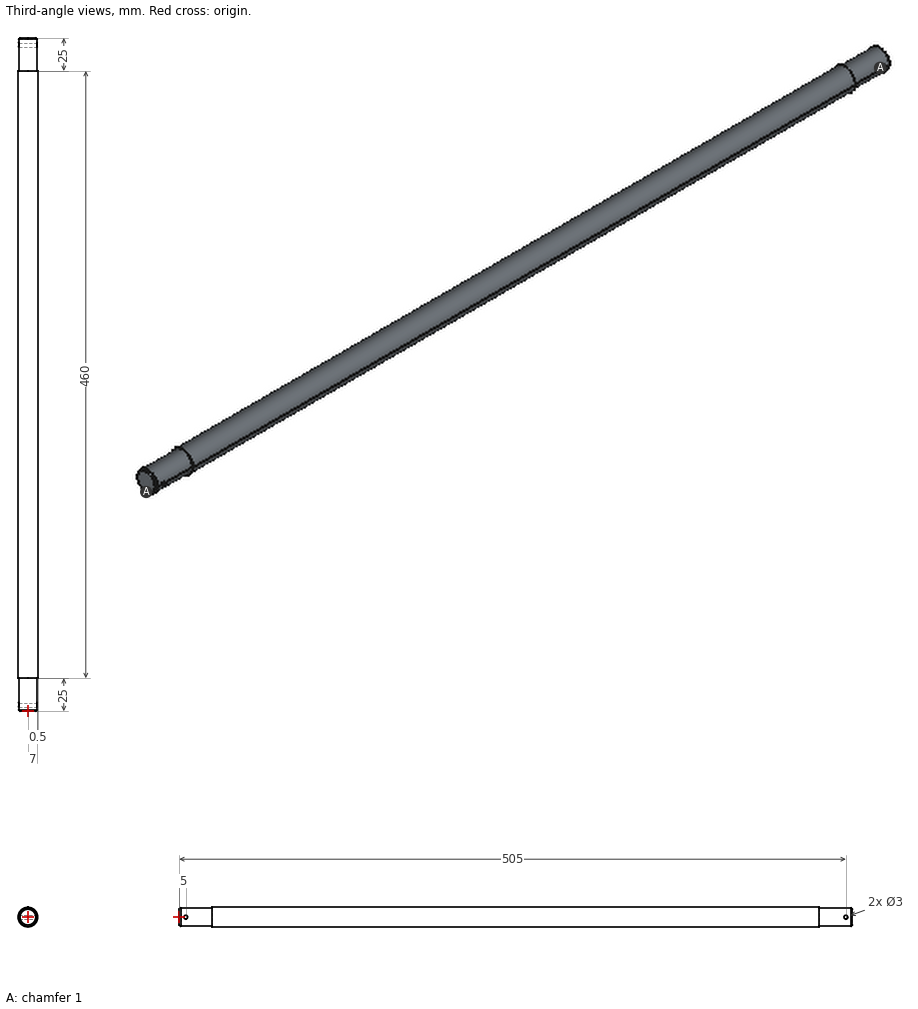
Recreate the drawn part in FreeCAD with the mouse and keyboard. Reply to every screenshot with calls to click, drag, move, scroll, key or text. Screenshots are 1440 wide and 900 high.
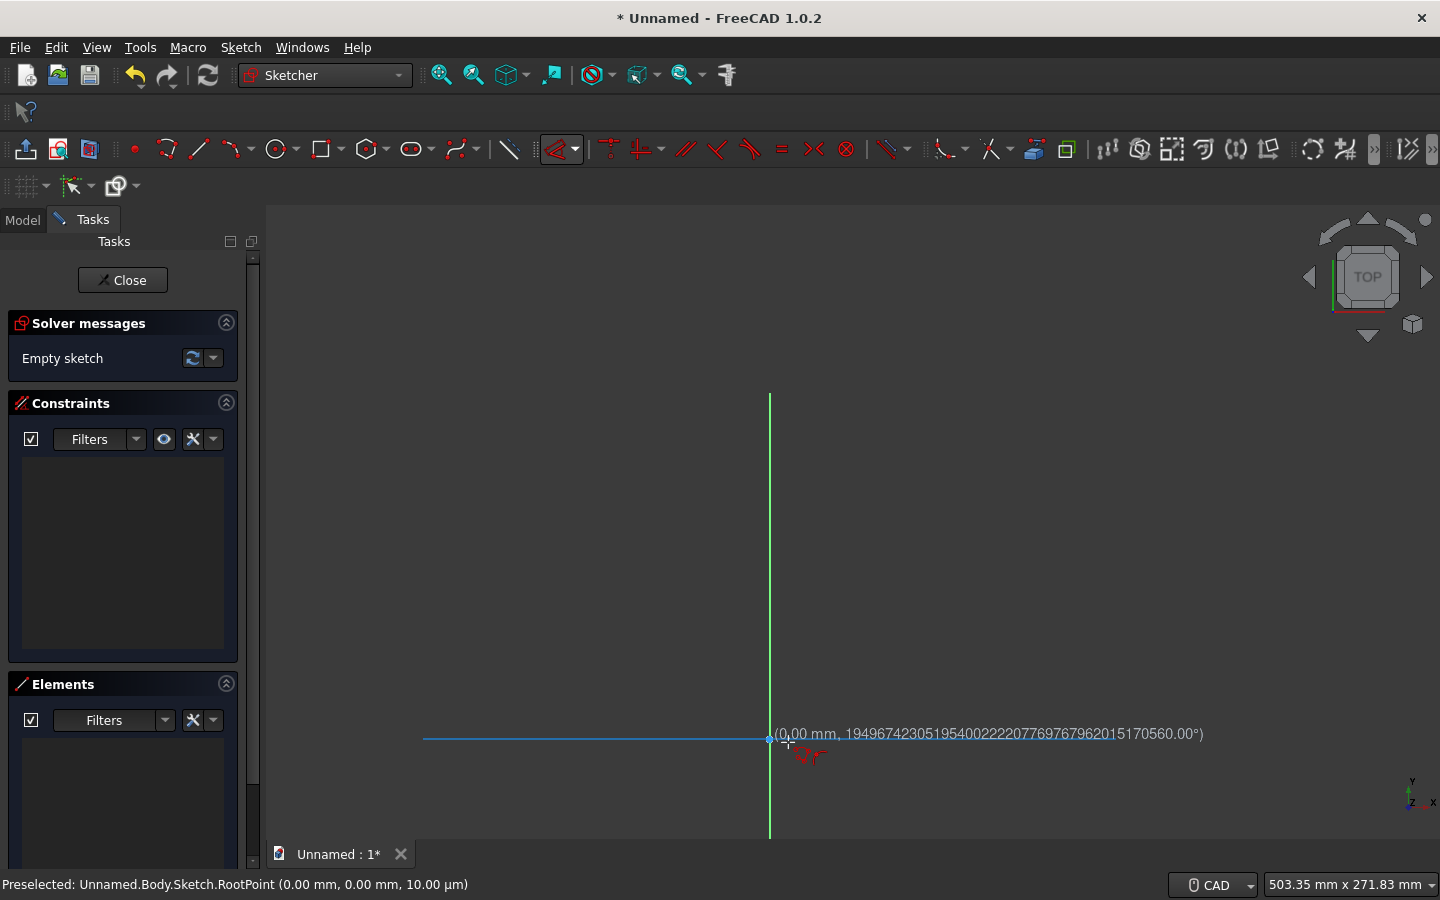
click(786, 730)
click(786, 681)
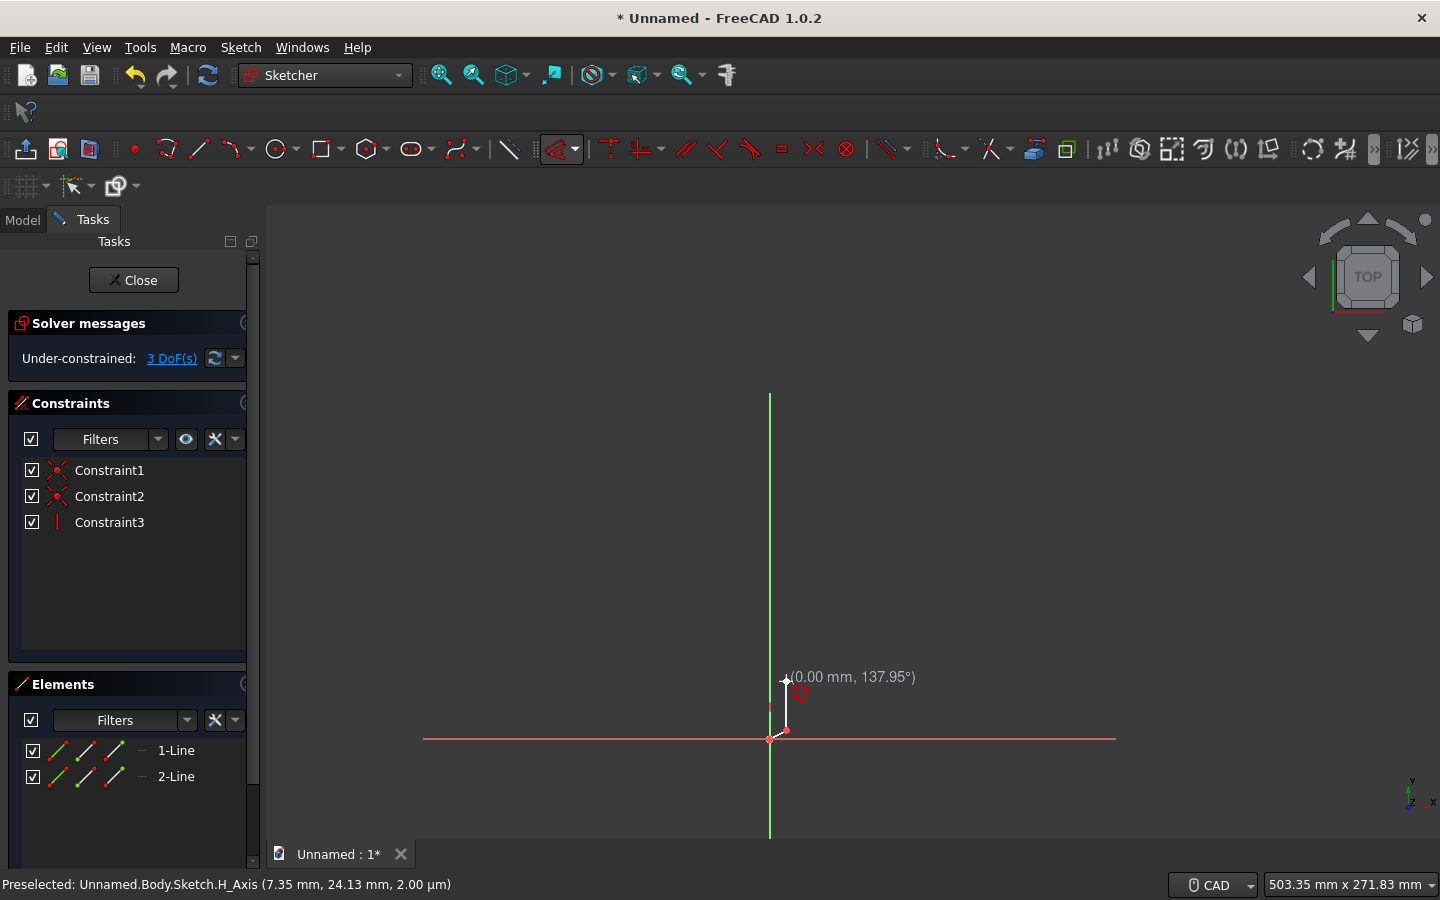
scroll(787, 681, up, 14)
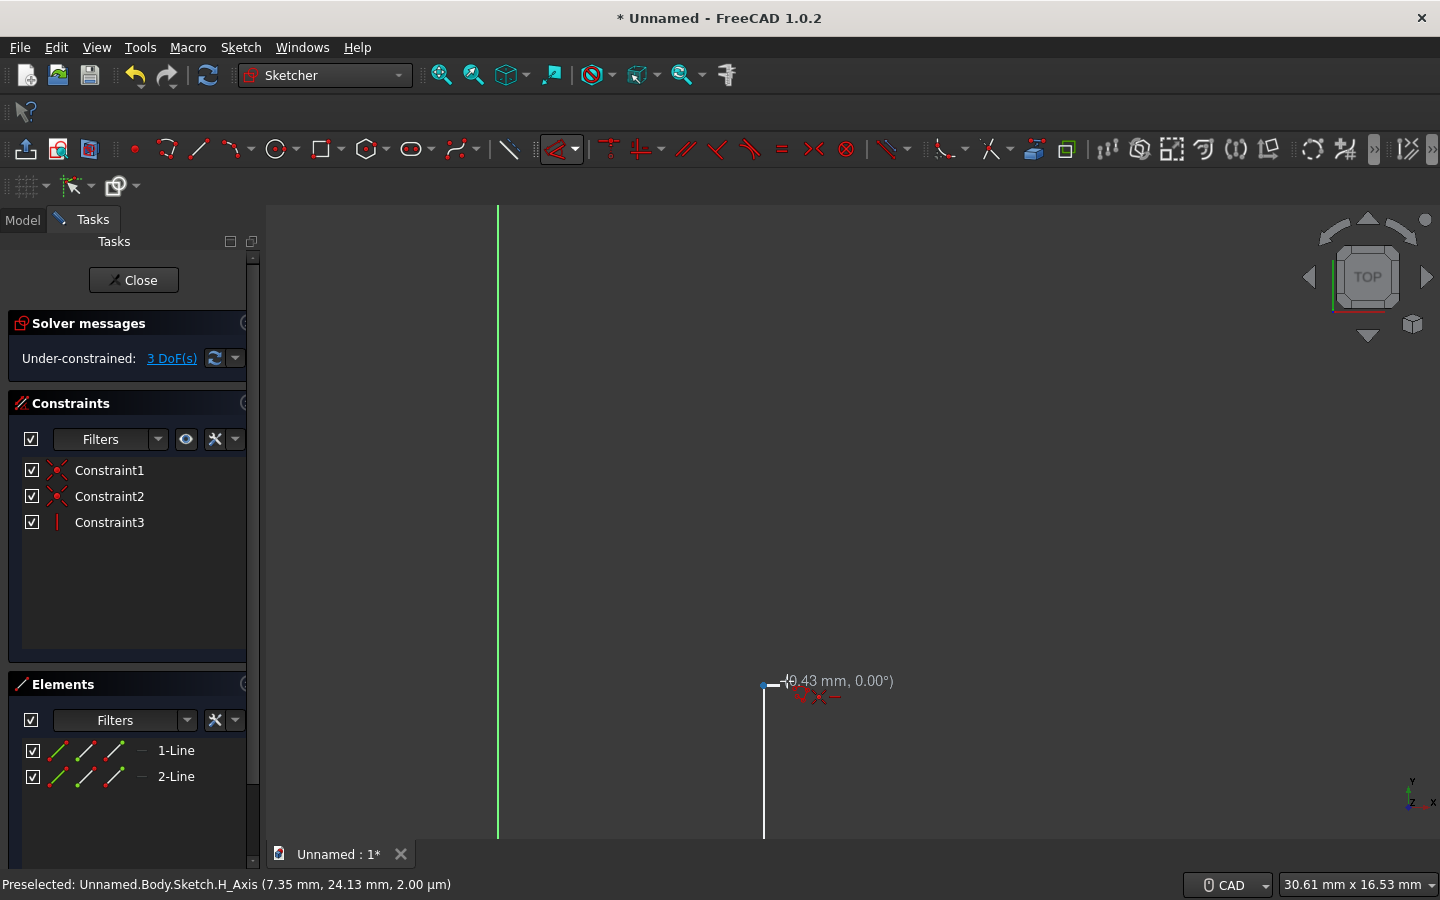
click(786, 669)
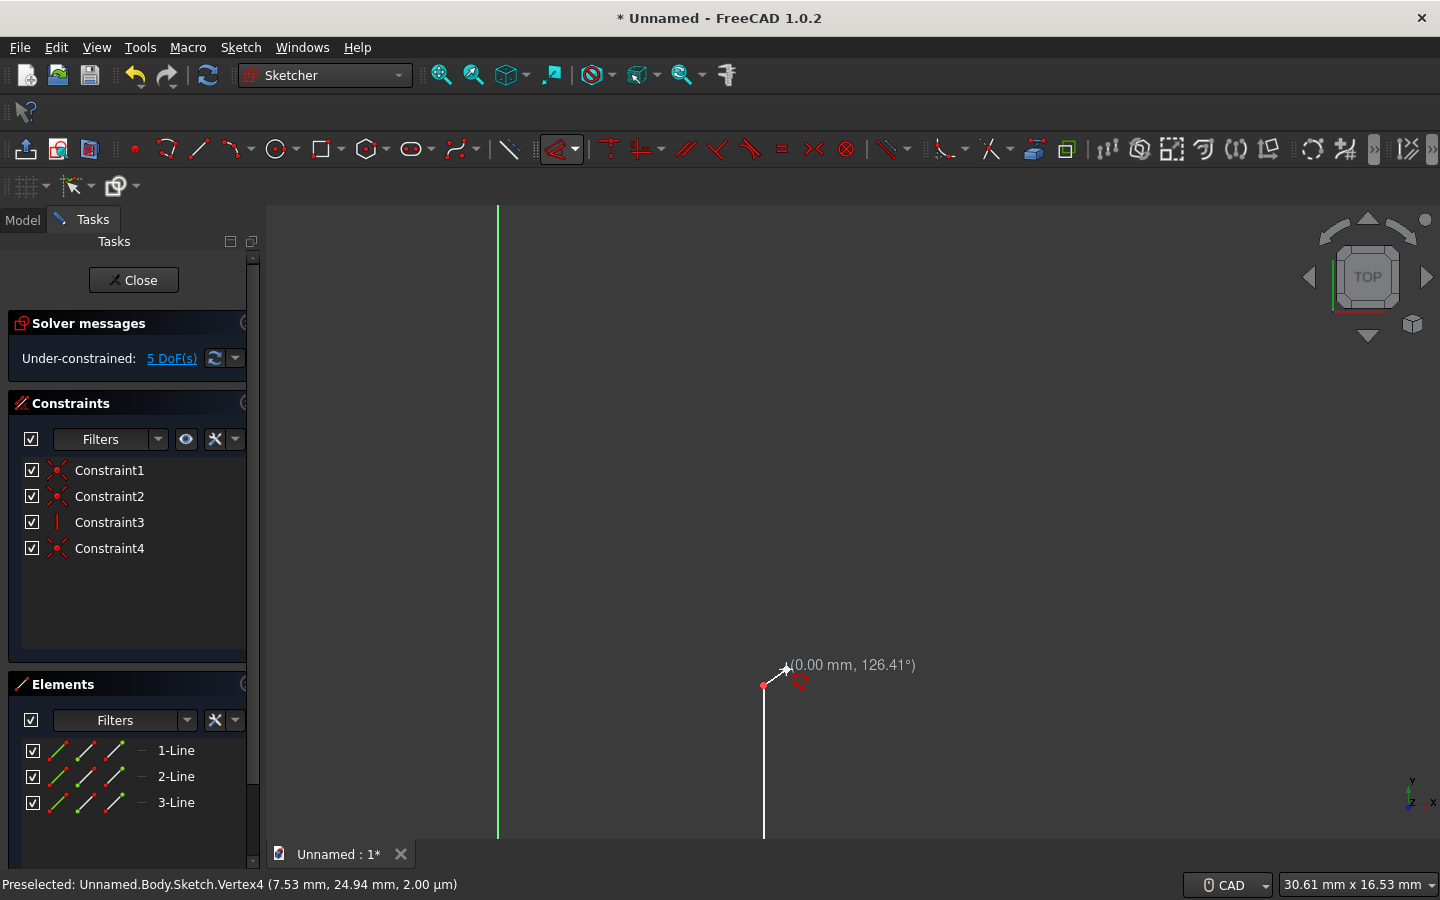
scroll(784, 522, down, 15)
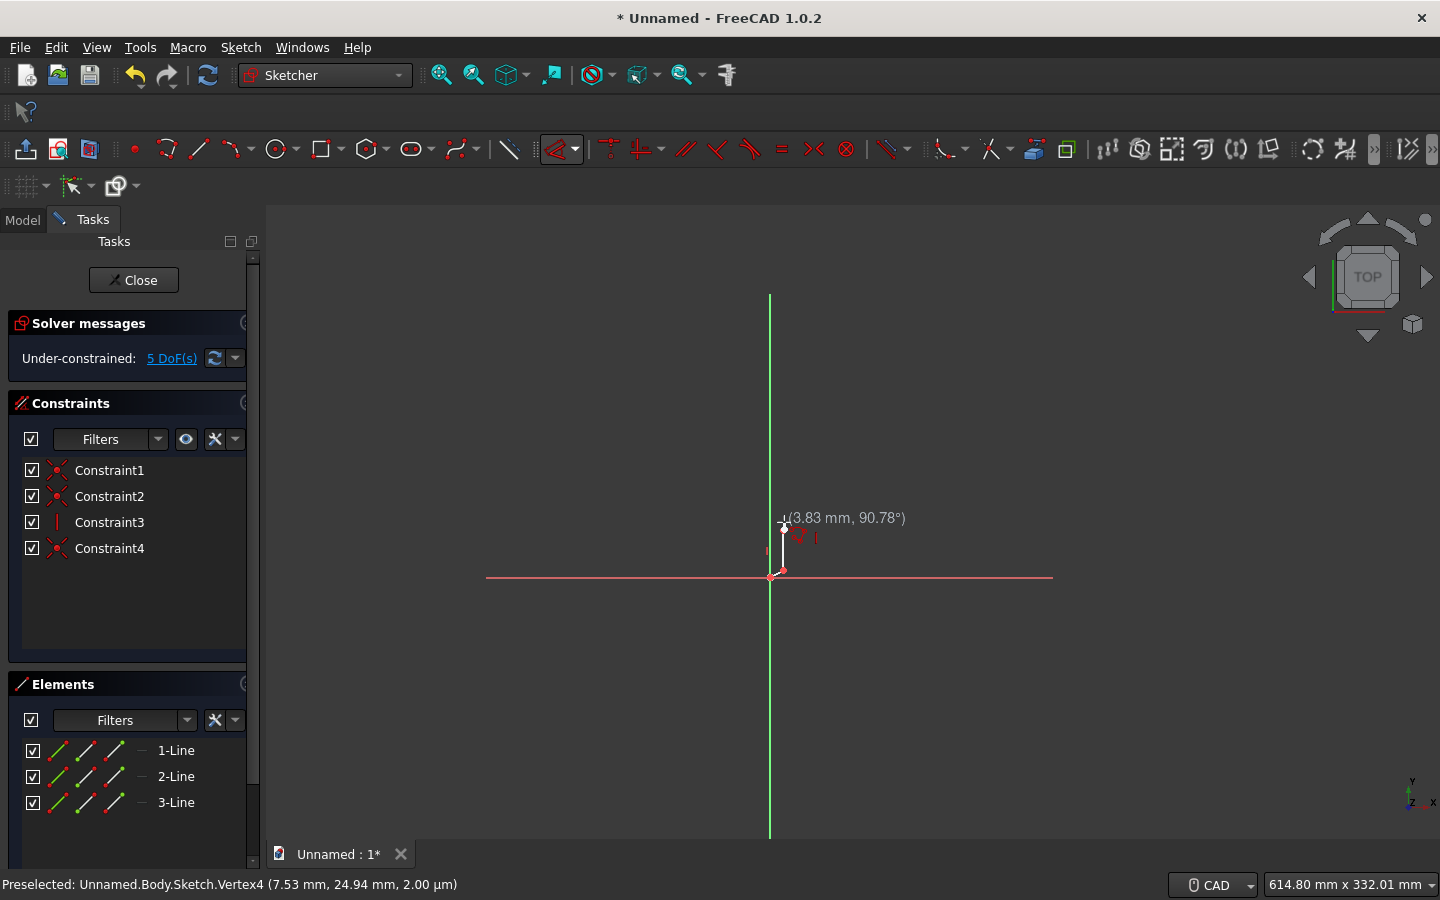
scroll(790, 811, down, 4)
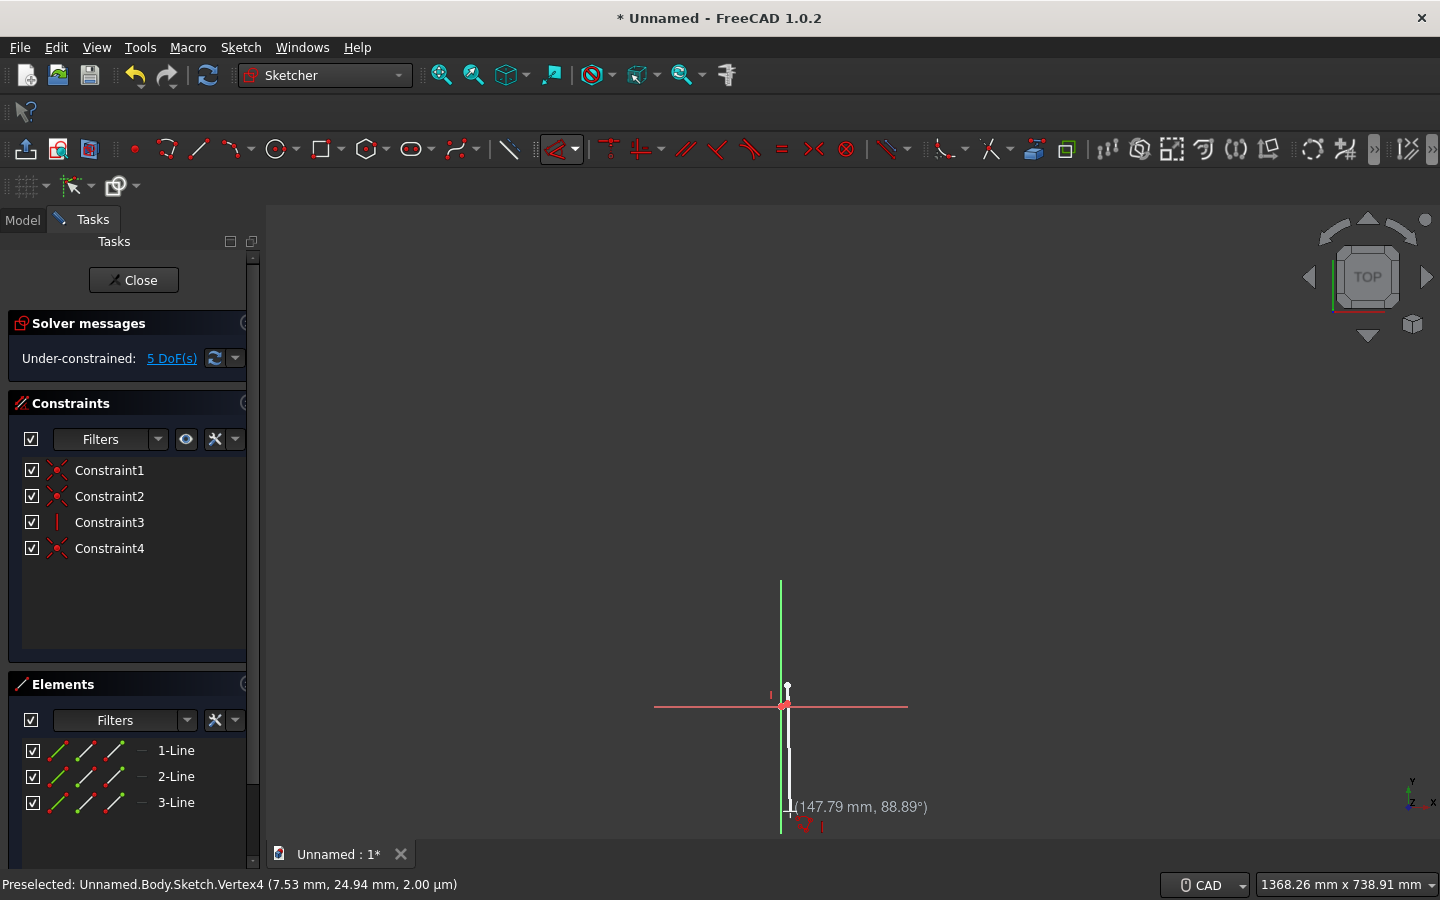
scroll(788, 290, up, 5)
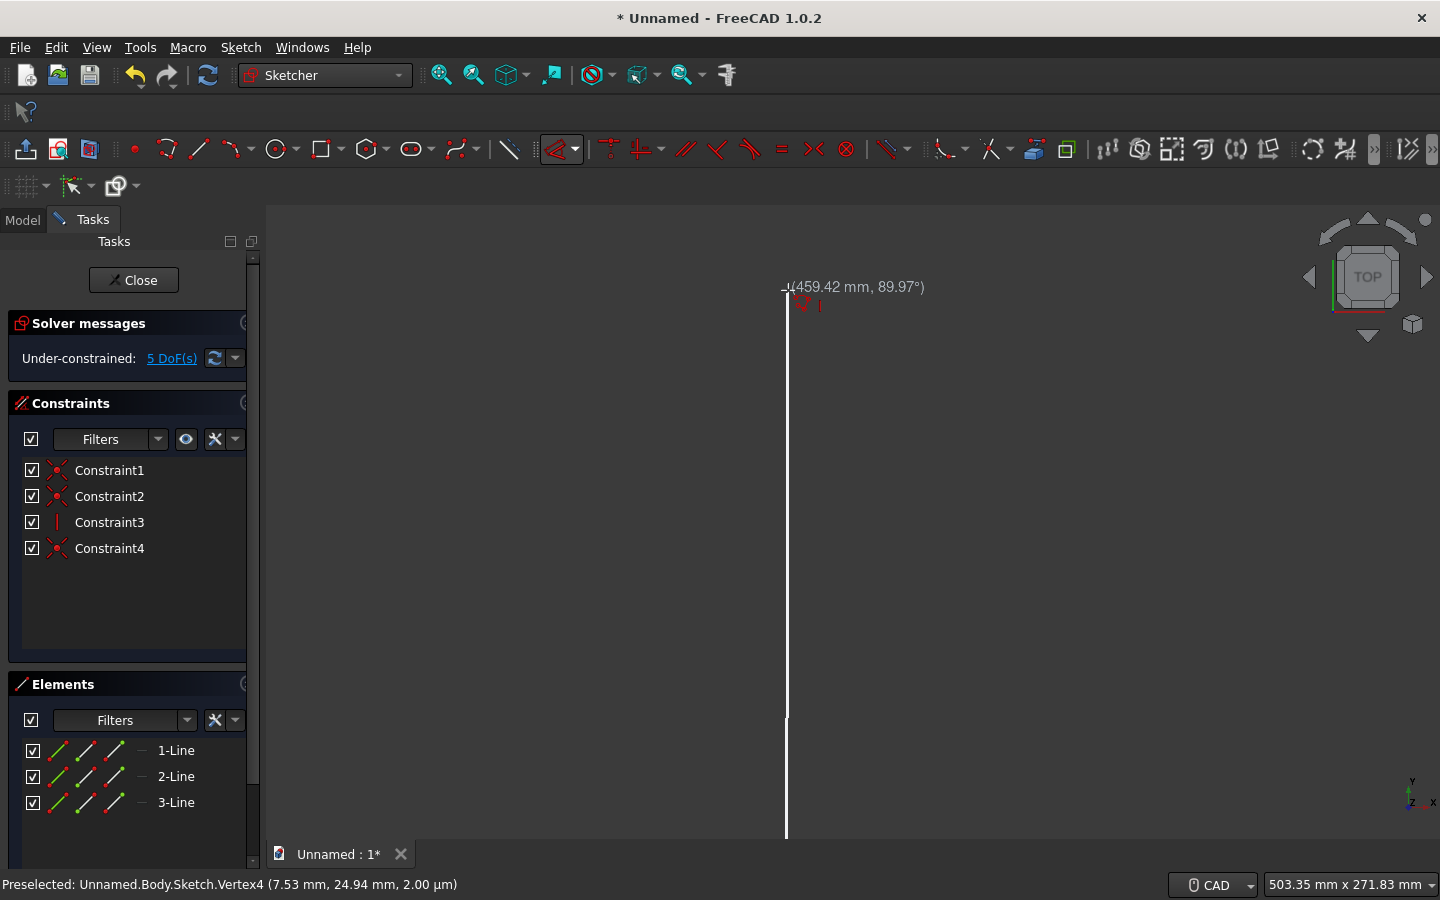
click(787, 291)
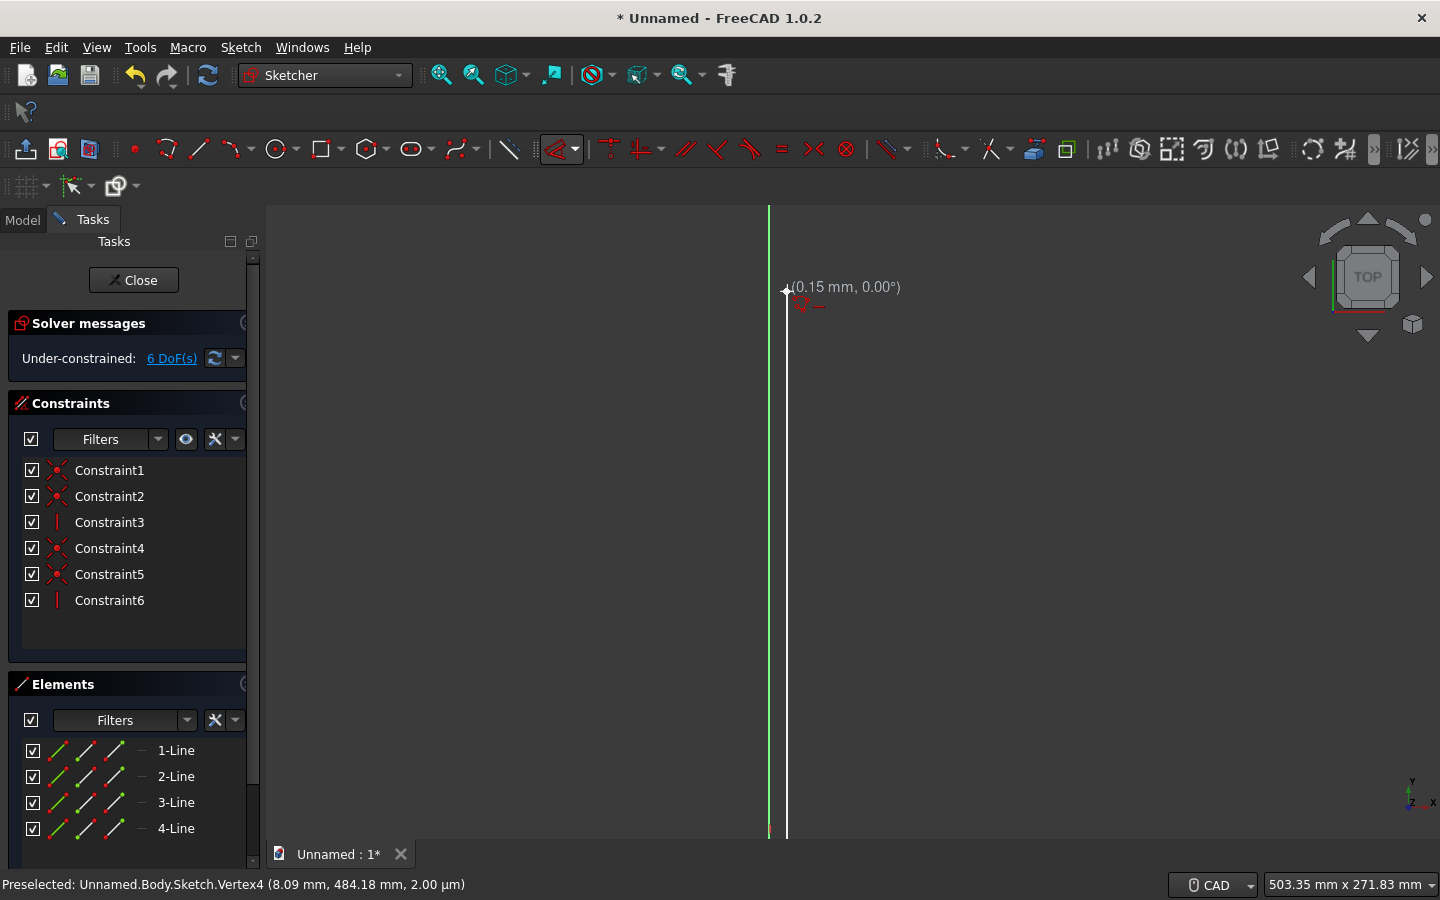
scroll(785, 291, up, 14)